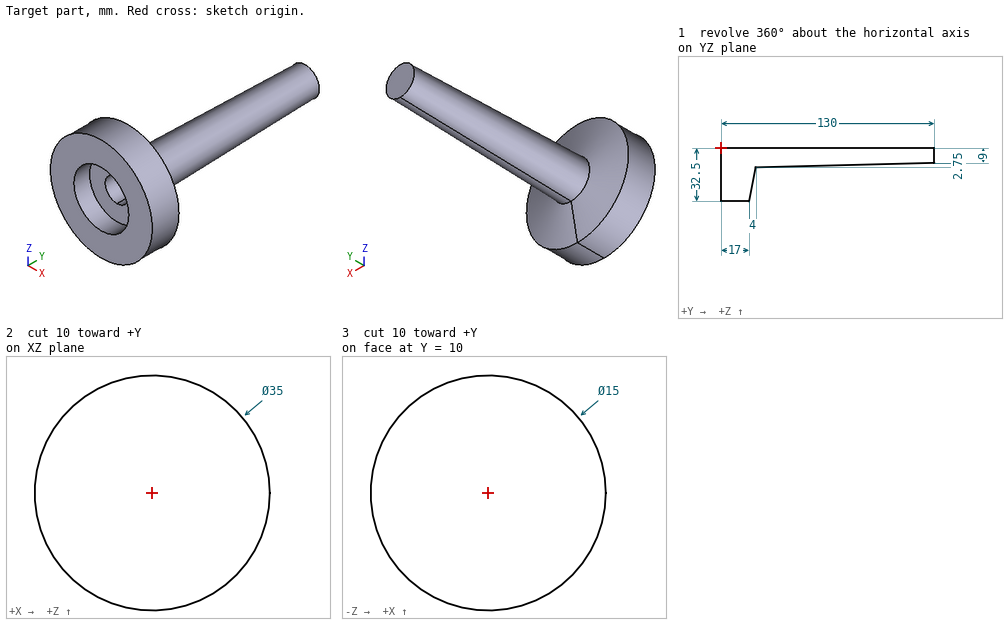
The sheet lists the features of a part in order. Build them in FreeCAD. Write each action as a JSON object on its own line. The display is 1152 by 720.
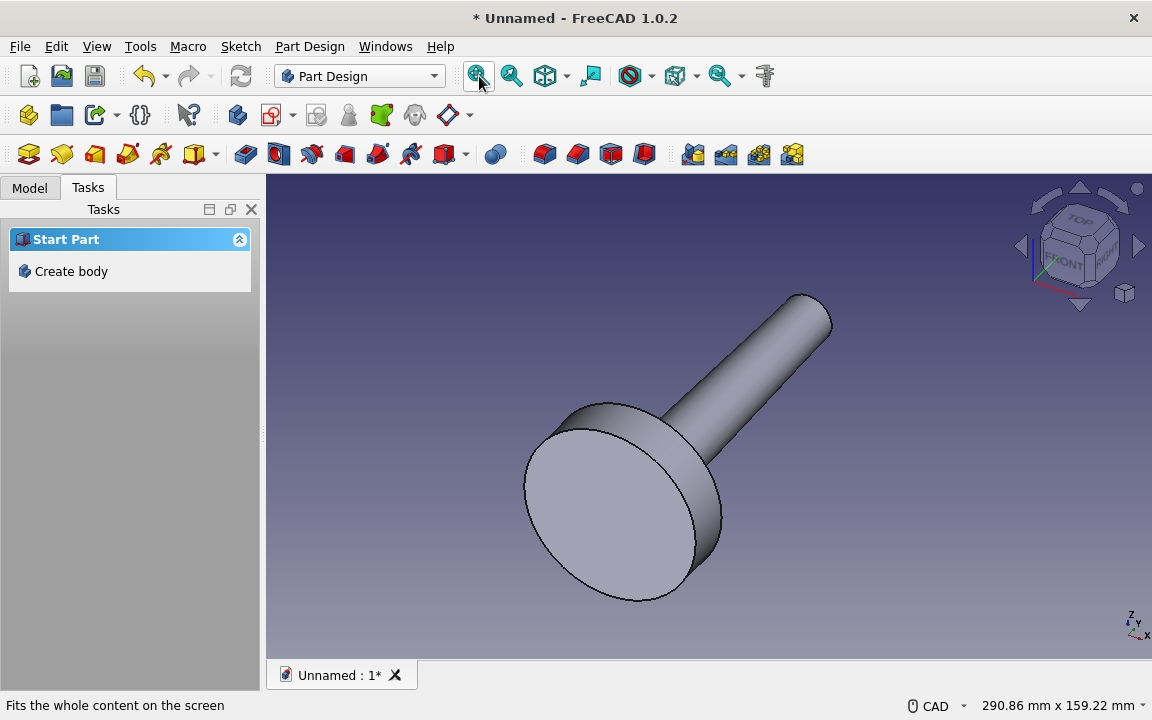
{"action": "left_click", "coordinate": [270, 116]}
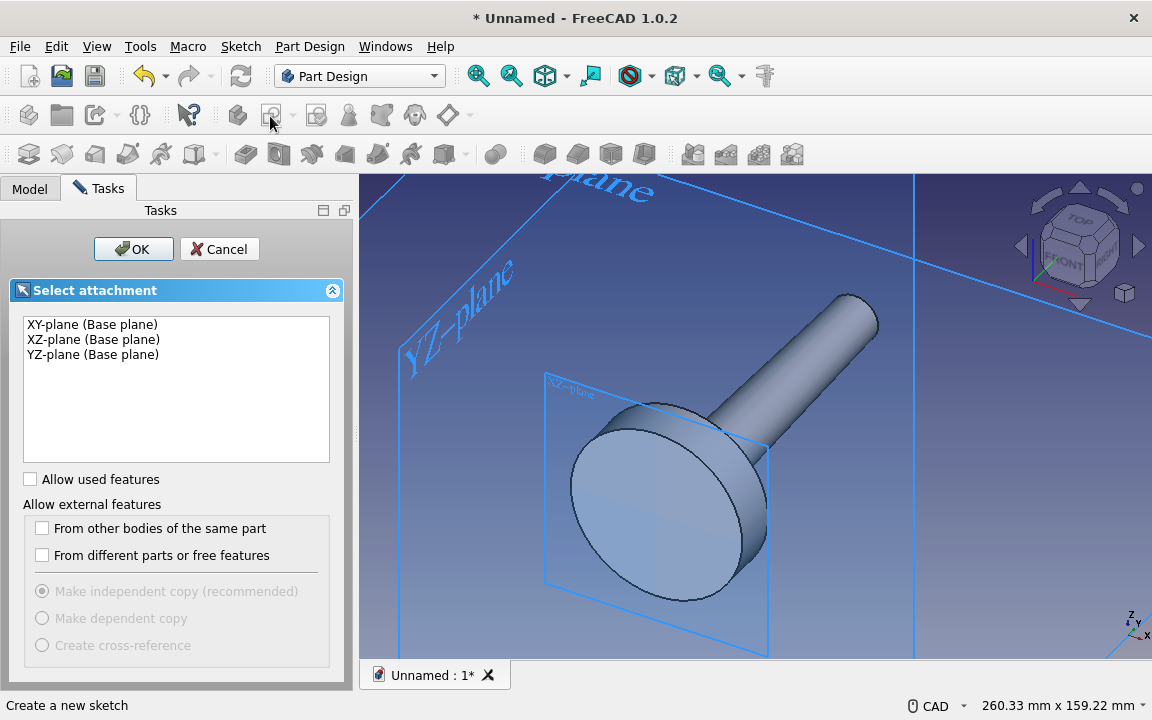
{"action": "left_click", "coordinate": [84, 340]}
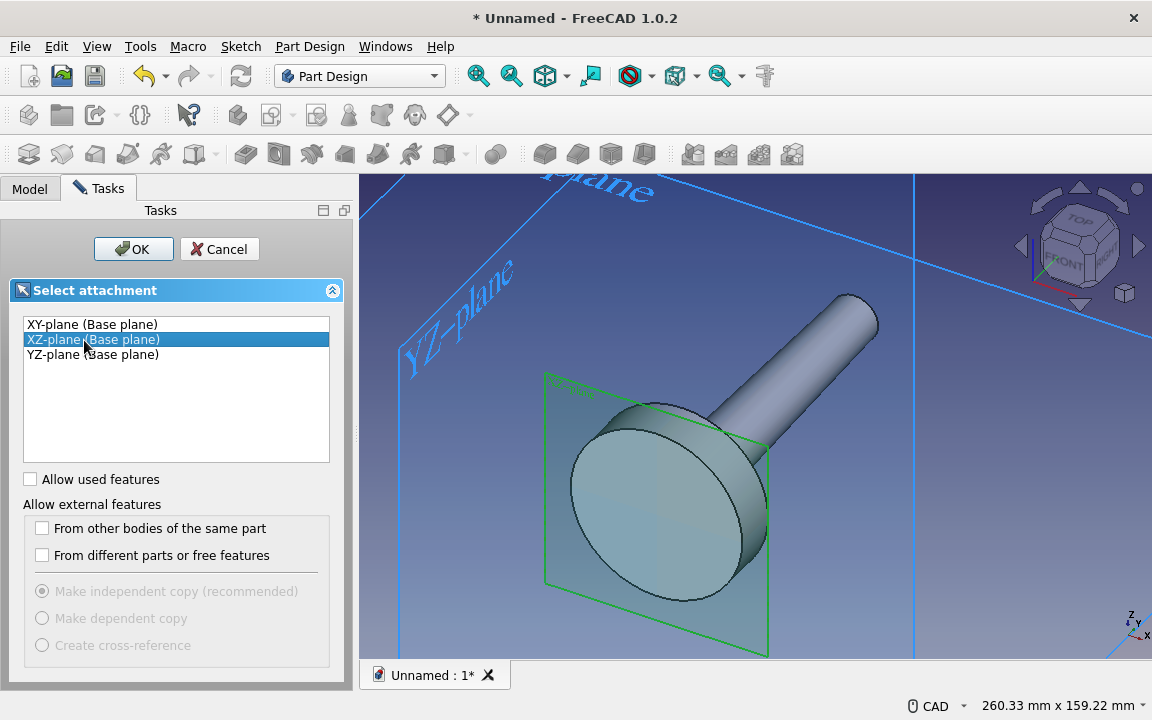
{"action": "left_click", "coordinate": [134, 249]}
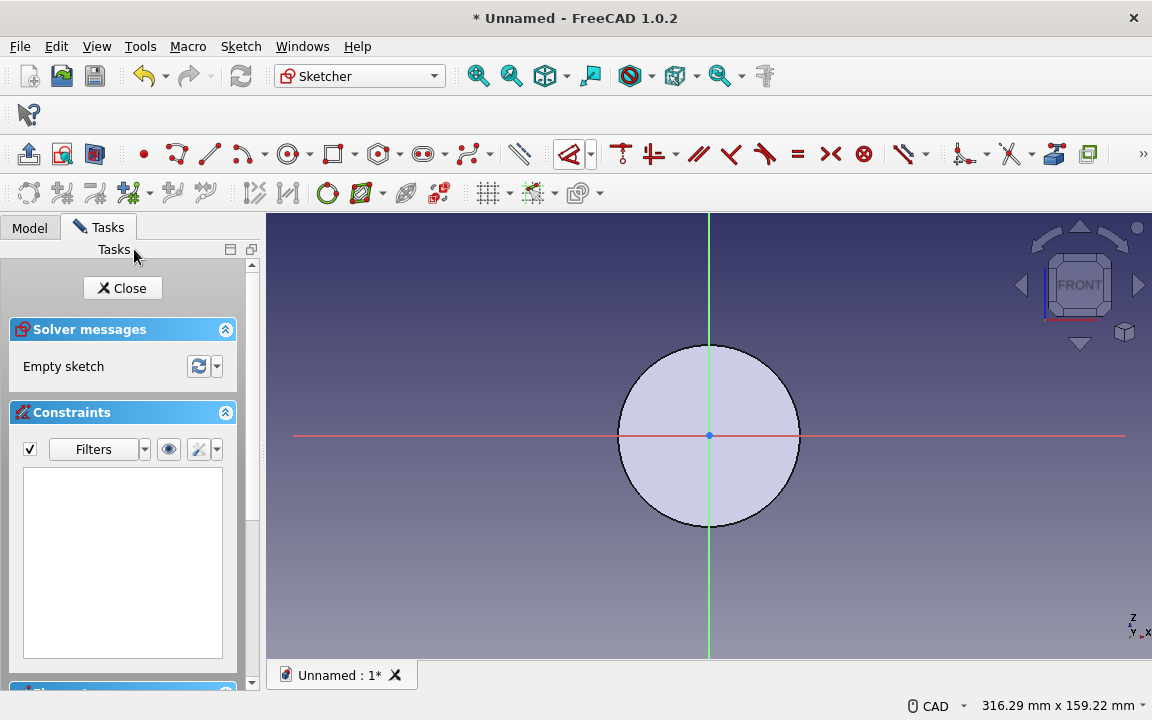
{"action": "scroll", "coordinate": [749, 436], "scroll_direction": "up", "scroll_amount": 5}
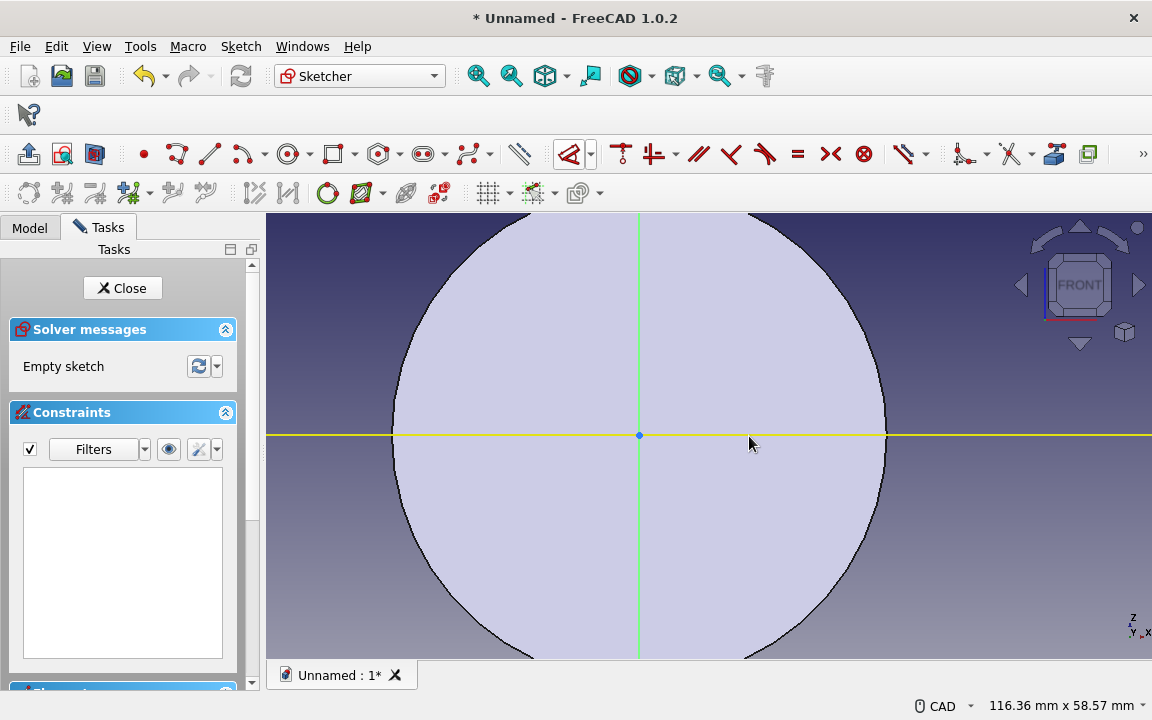
{"action": "left_click", "coordinate": [288, 154]}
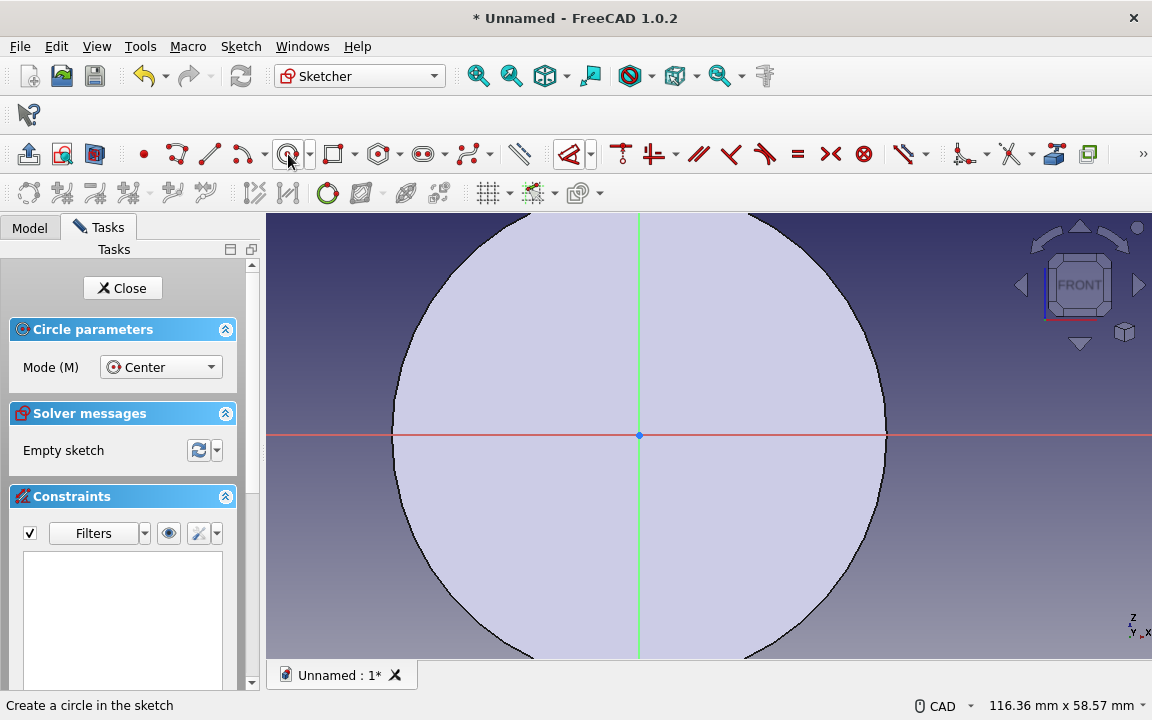
{"action": "left_click", "coordinate": [639, 435]}
{"action": "mouse_move", "coordinate": [734, 341]}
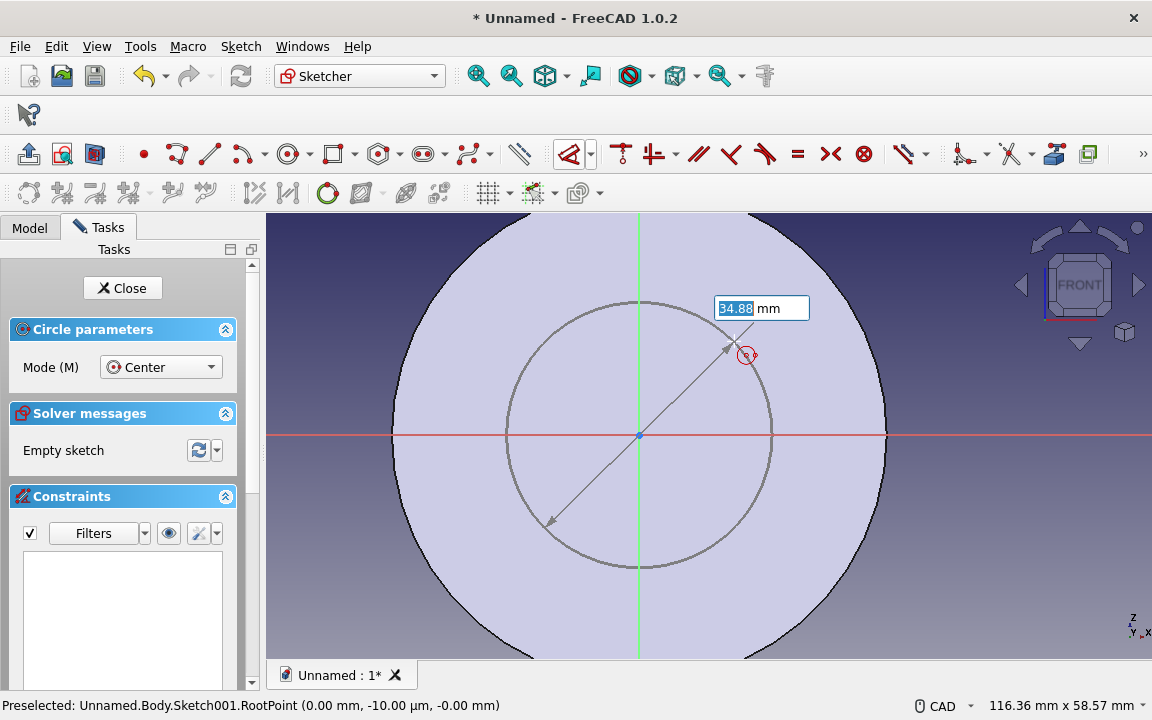
{"action": "type", "text": "35"}
{"action": "key", "text": "Return"}
{"action": "key", "text": "Escape"}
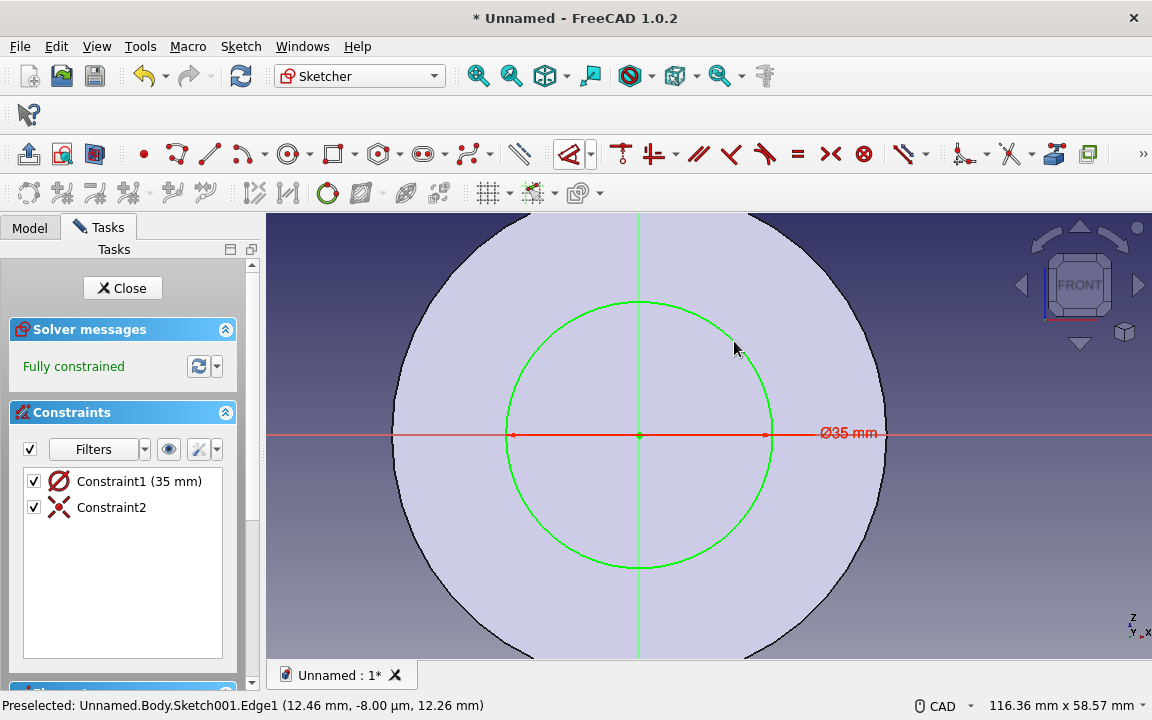
{"action": "left_click", "coordinate": [123, 288]}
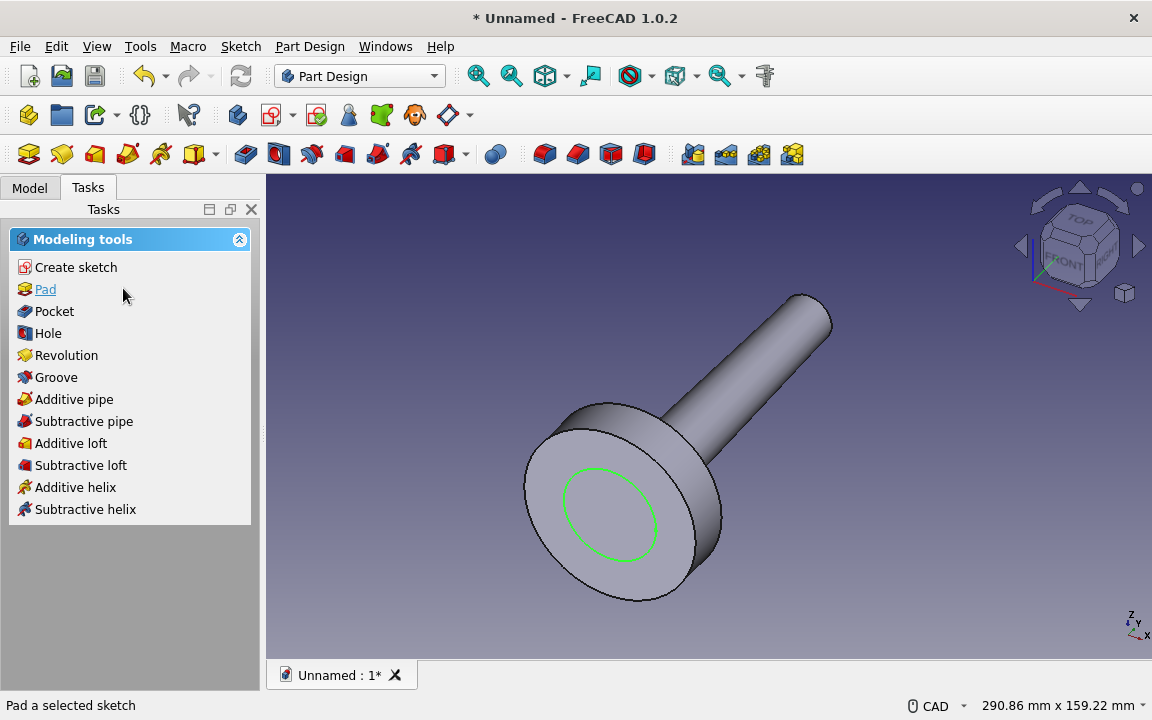
{"action": "left_click", "coordinate": [246, 154]}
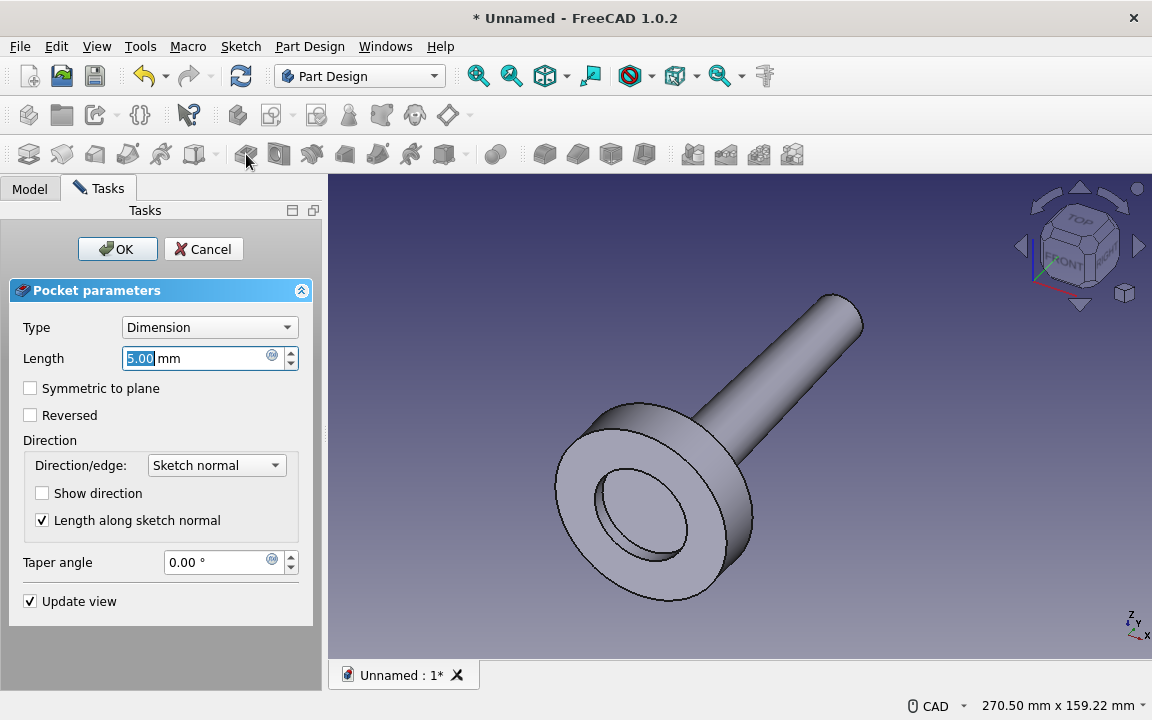
{"action": "type", "text": "10"}
{"action": "key", "text": "Tab"}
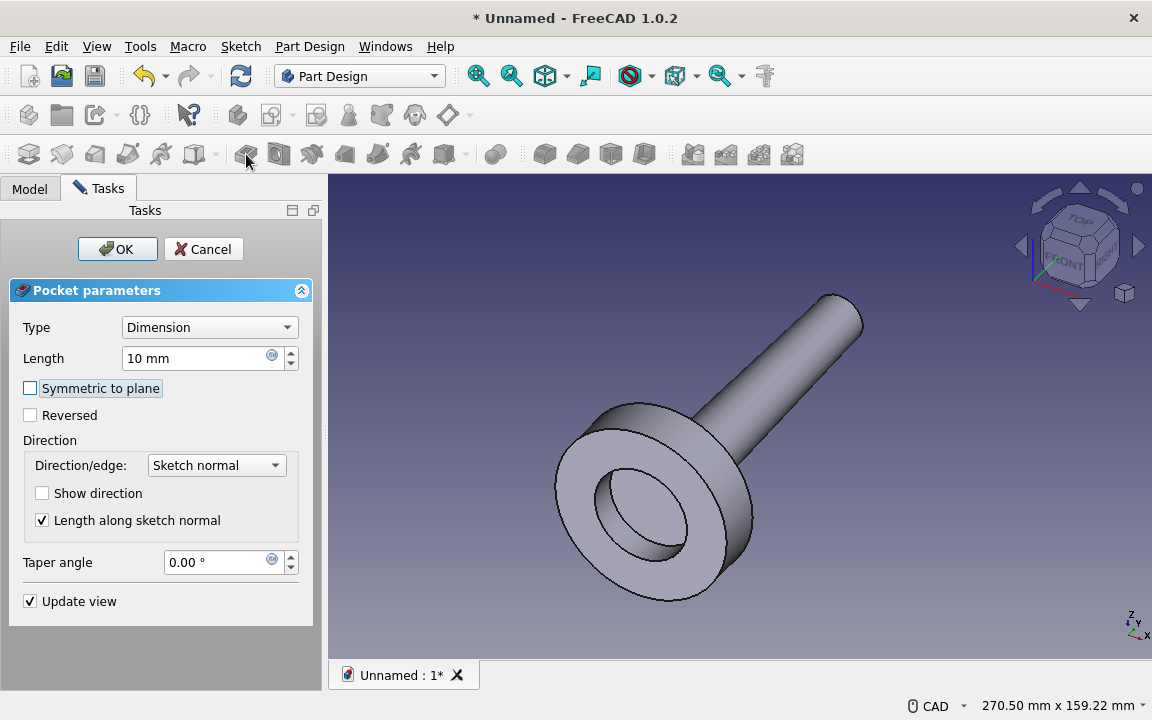
{"action": "left_click", "coordinate": [118, 249]}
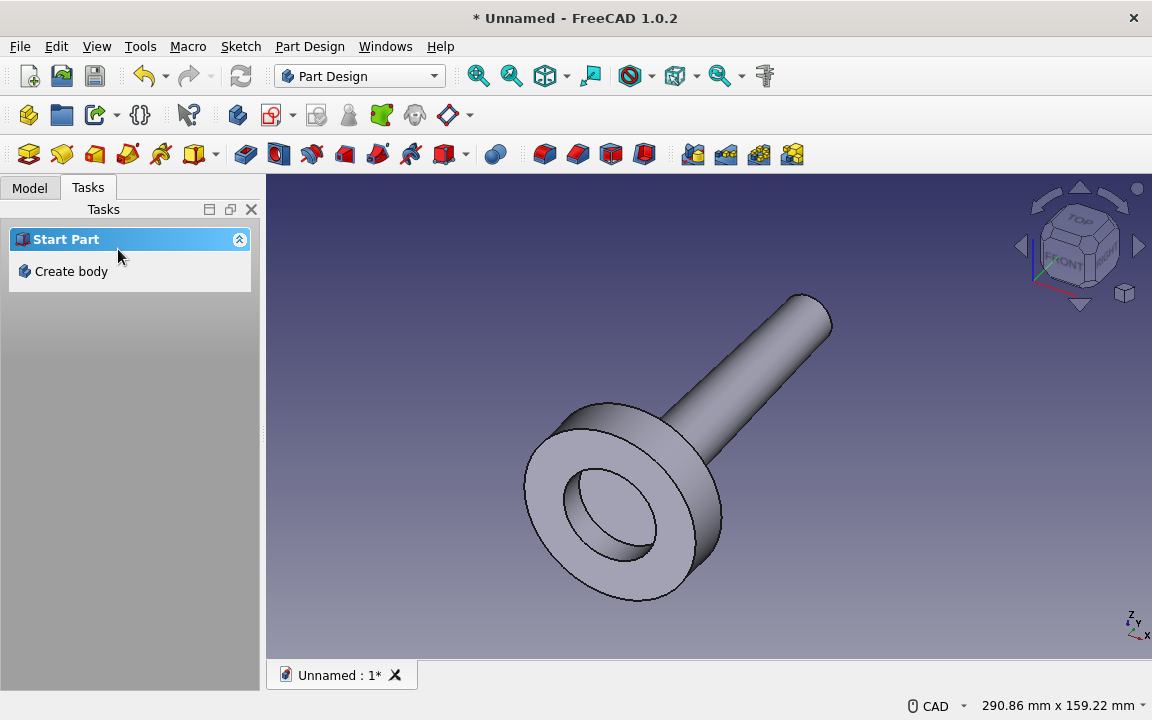
{"action": "left_click", "coordinate": [625, 499]}